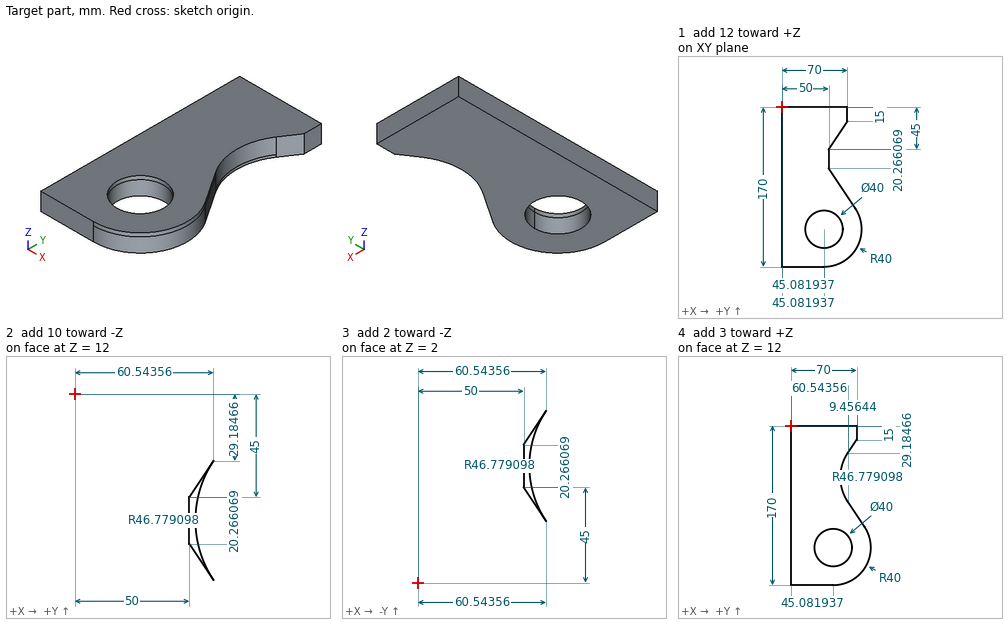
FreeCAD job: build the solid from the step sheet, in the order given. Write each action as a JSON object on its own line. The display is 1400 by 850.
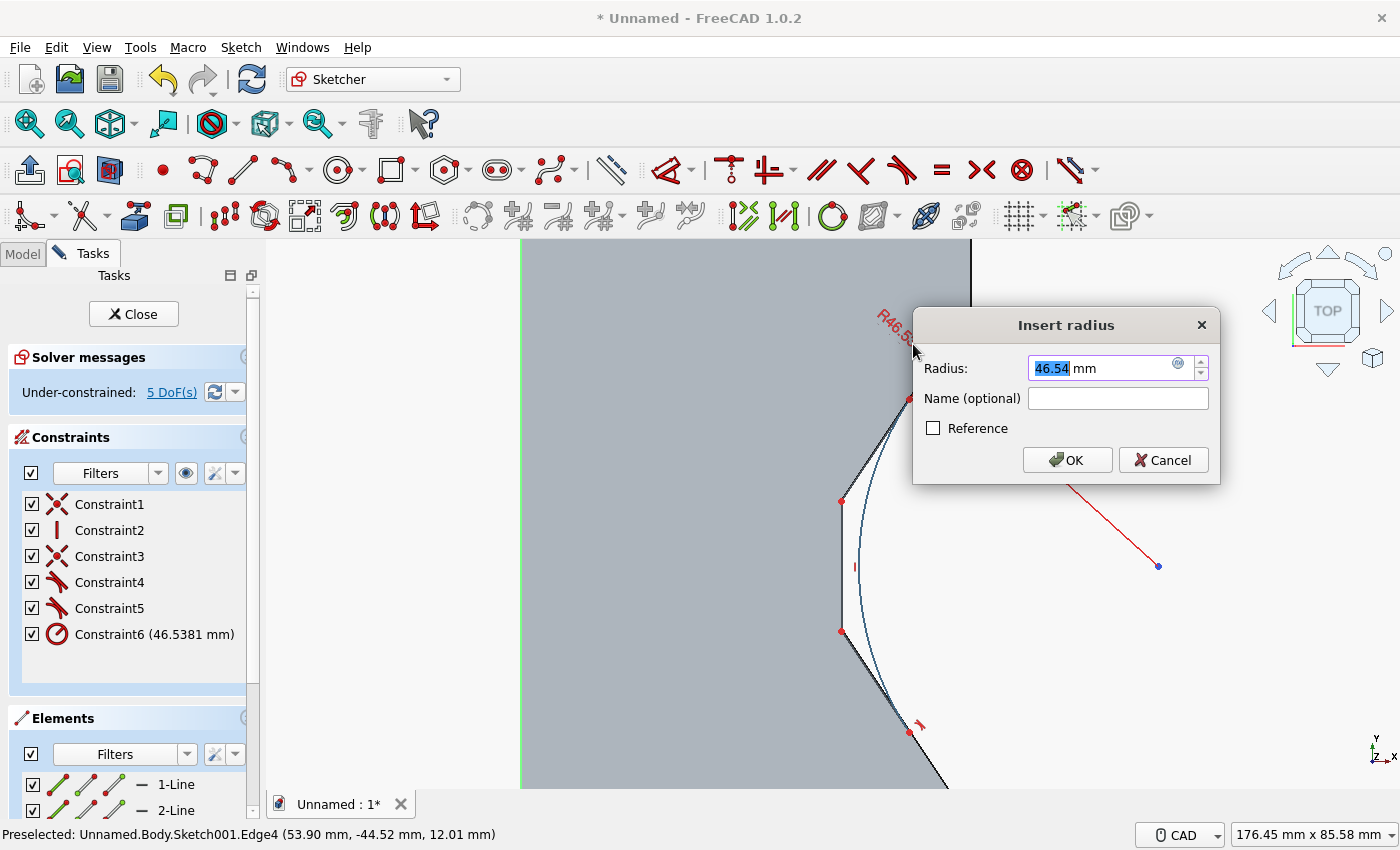
{"action": "type", "text": "46.779098"}
{"action": "key", "text": "Return"}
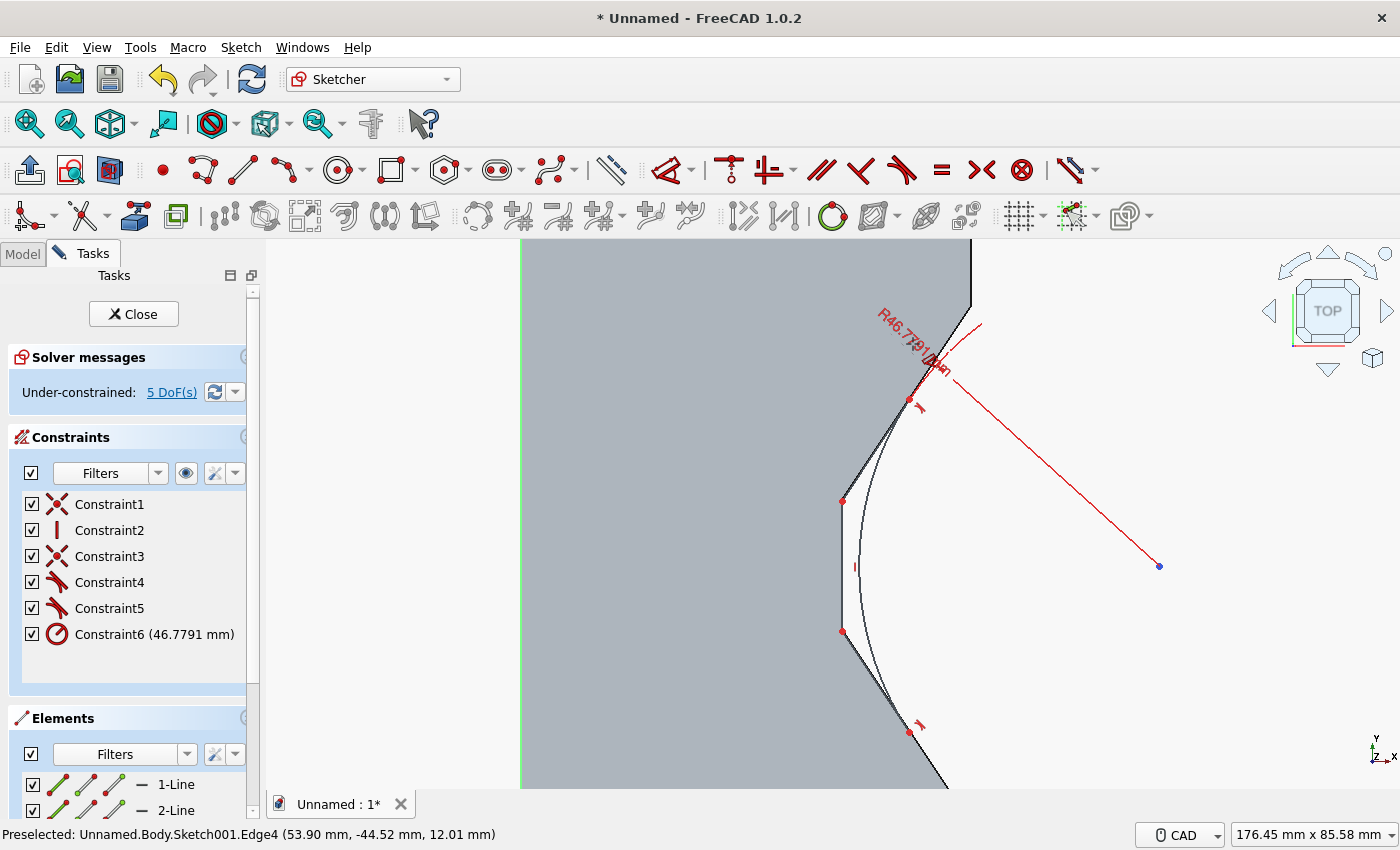
{"action": "left_click", "coordinate": [842, 501]}
{"action": "left_click", "coordinate": [681, 535]}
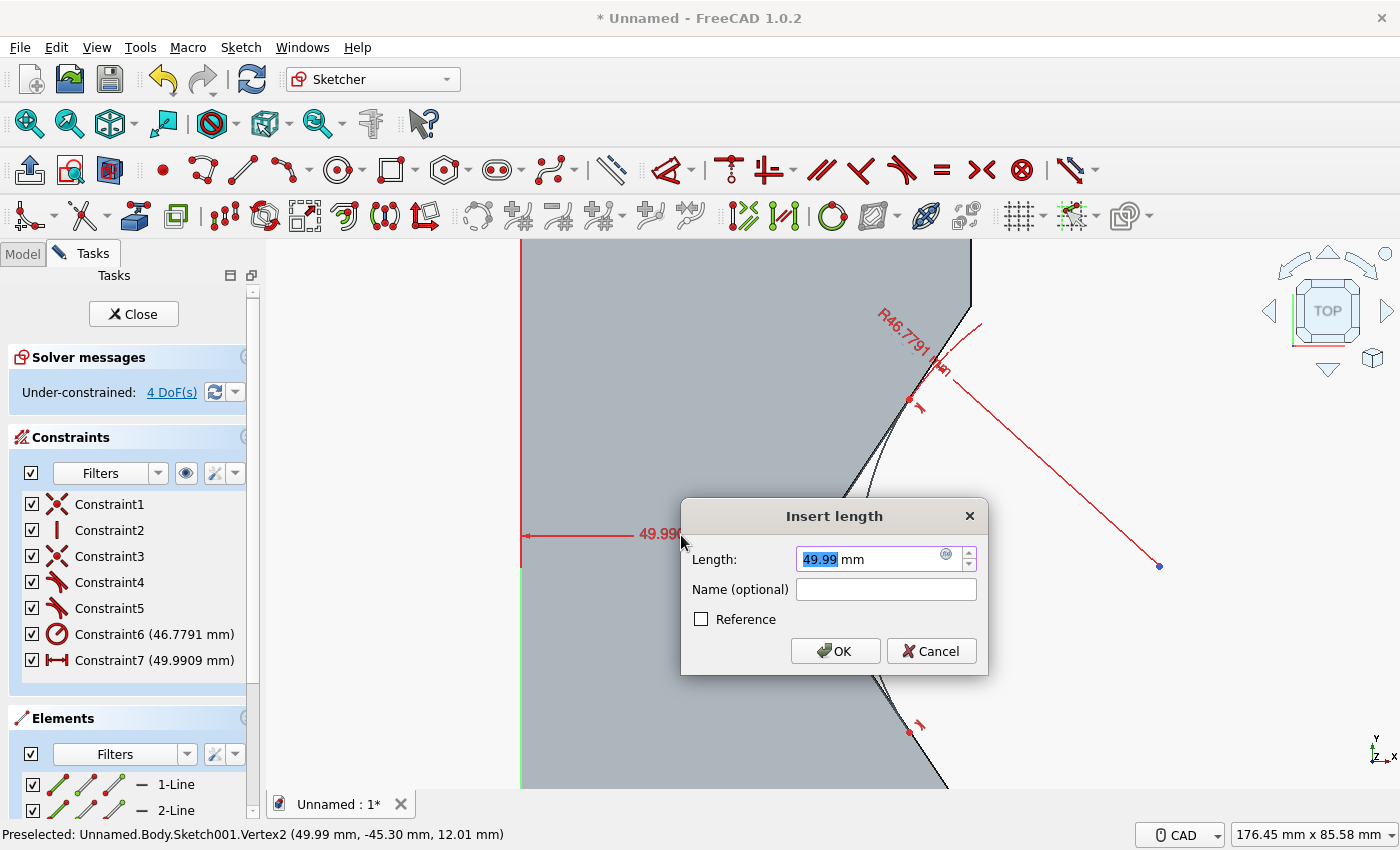
{"action": "type", "text": "50"}
{"action": "key", "text": "Return"}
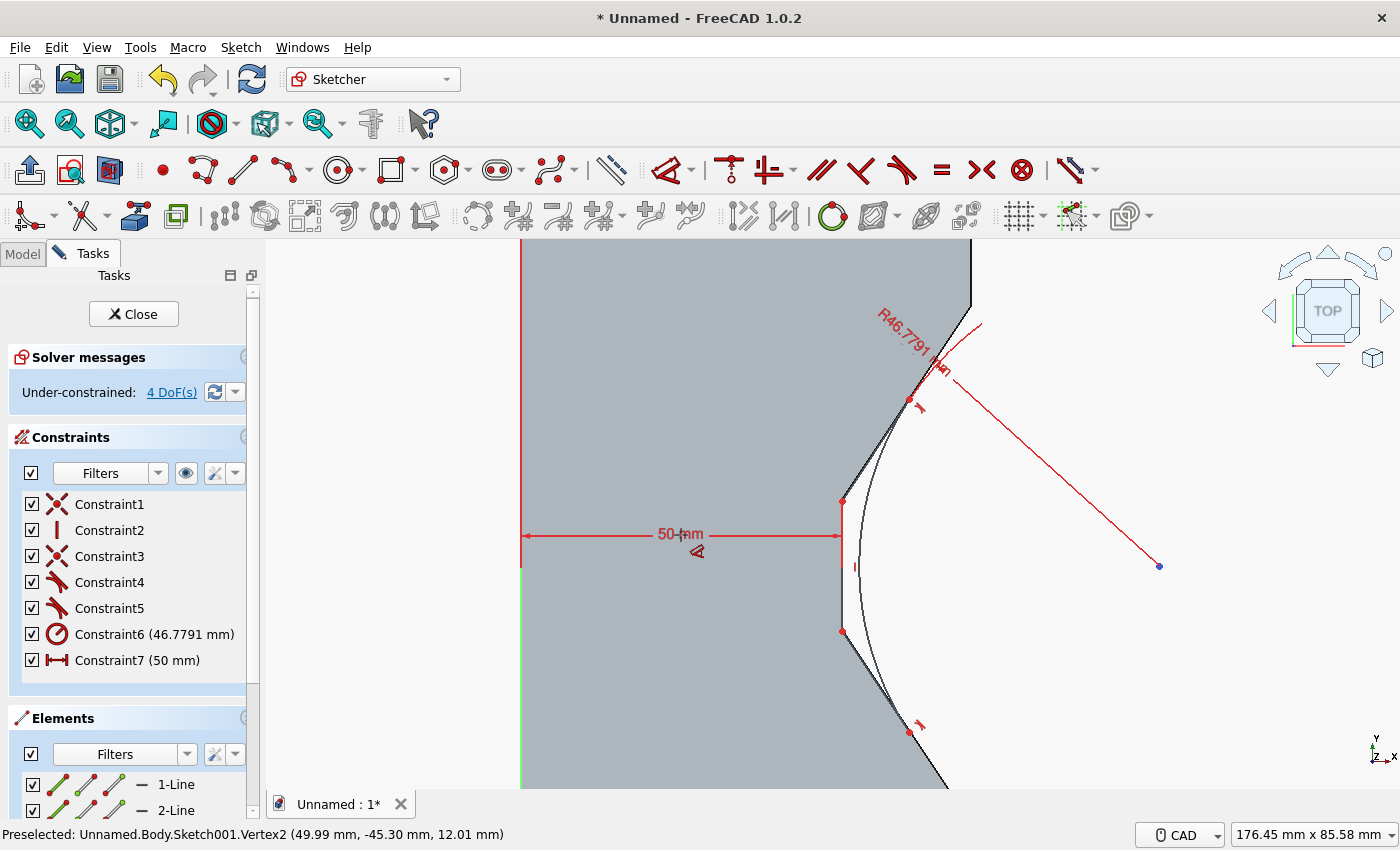
{"action": "left_click", "coordinate": [842, 501]}
{"action": "left_click", "coordinate": [487, 384]}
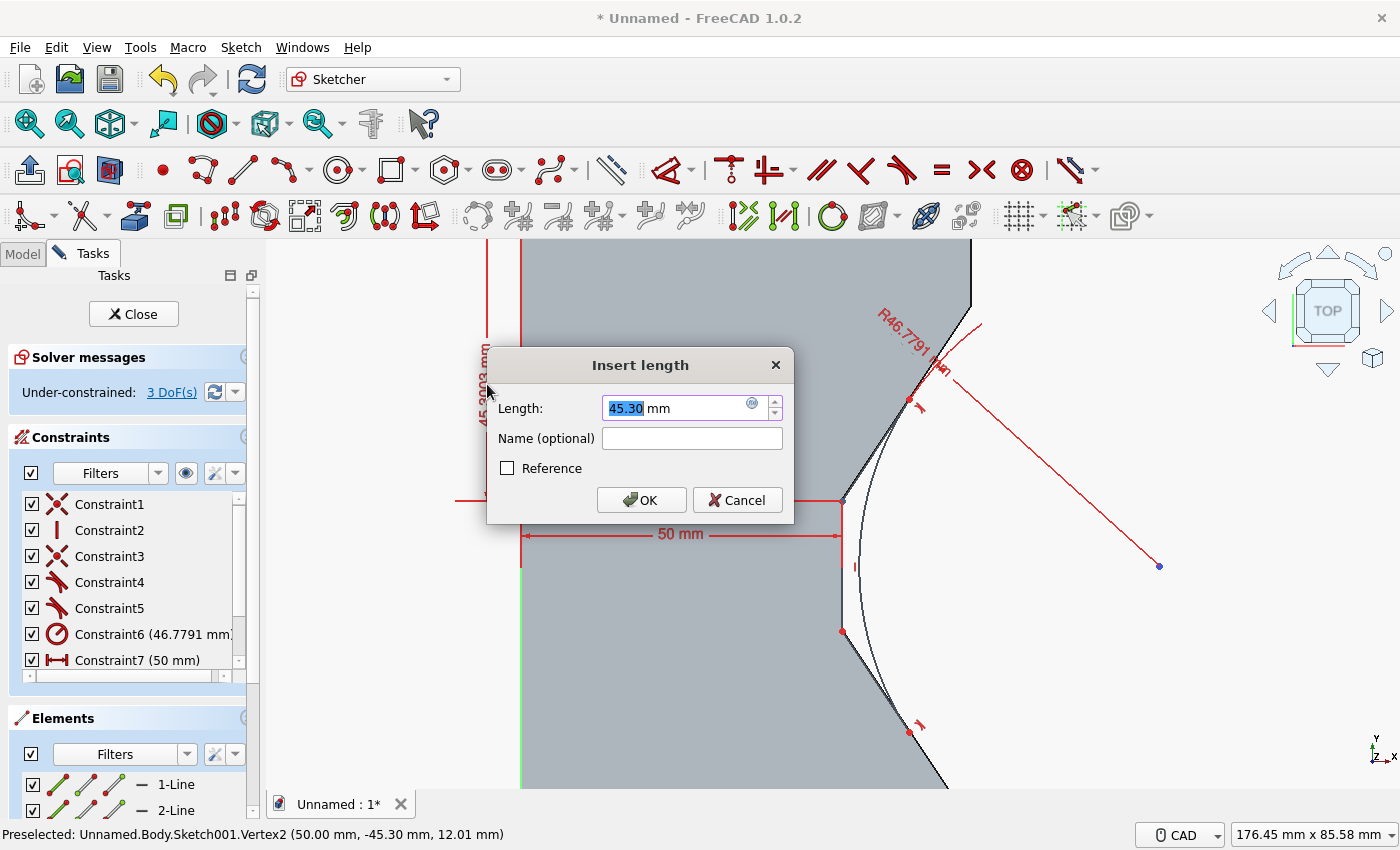
{"action": "type", "text": "45"}
{"action": "key", "text": "Return"}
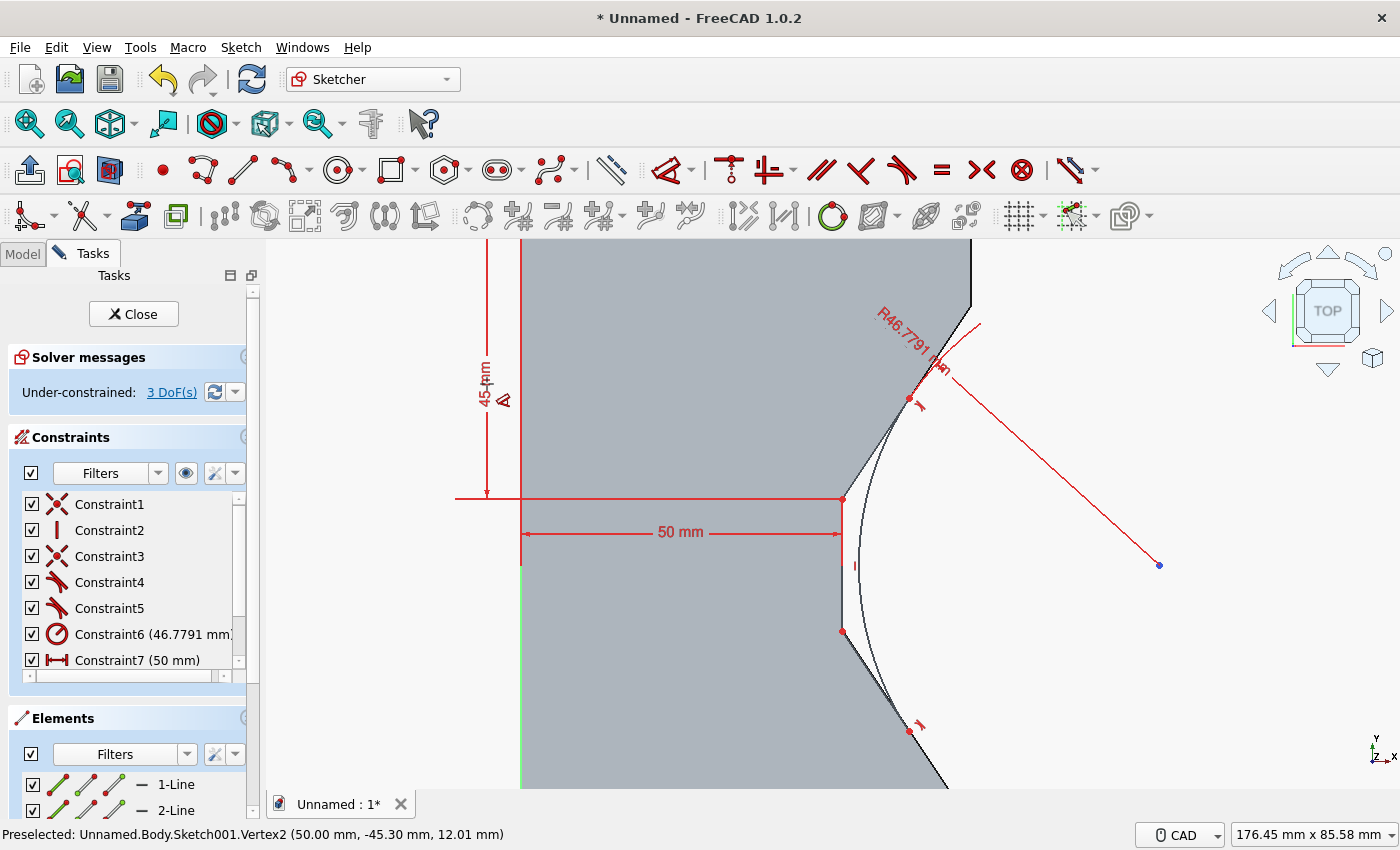
{"action": "left_click", "coordinate": [842, 539]}
{"action": "left_click", "coordinate": [876, 565]}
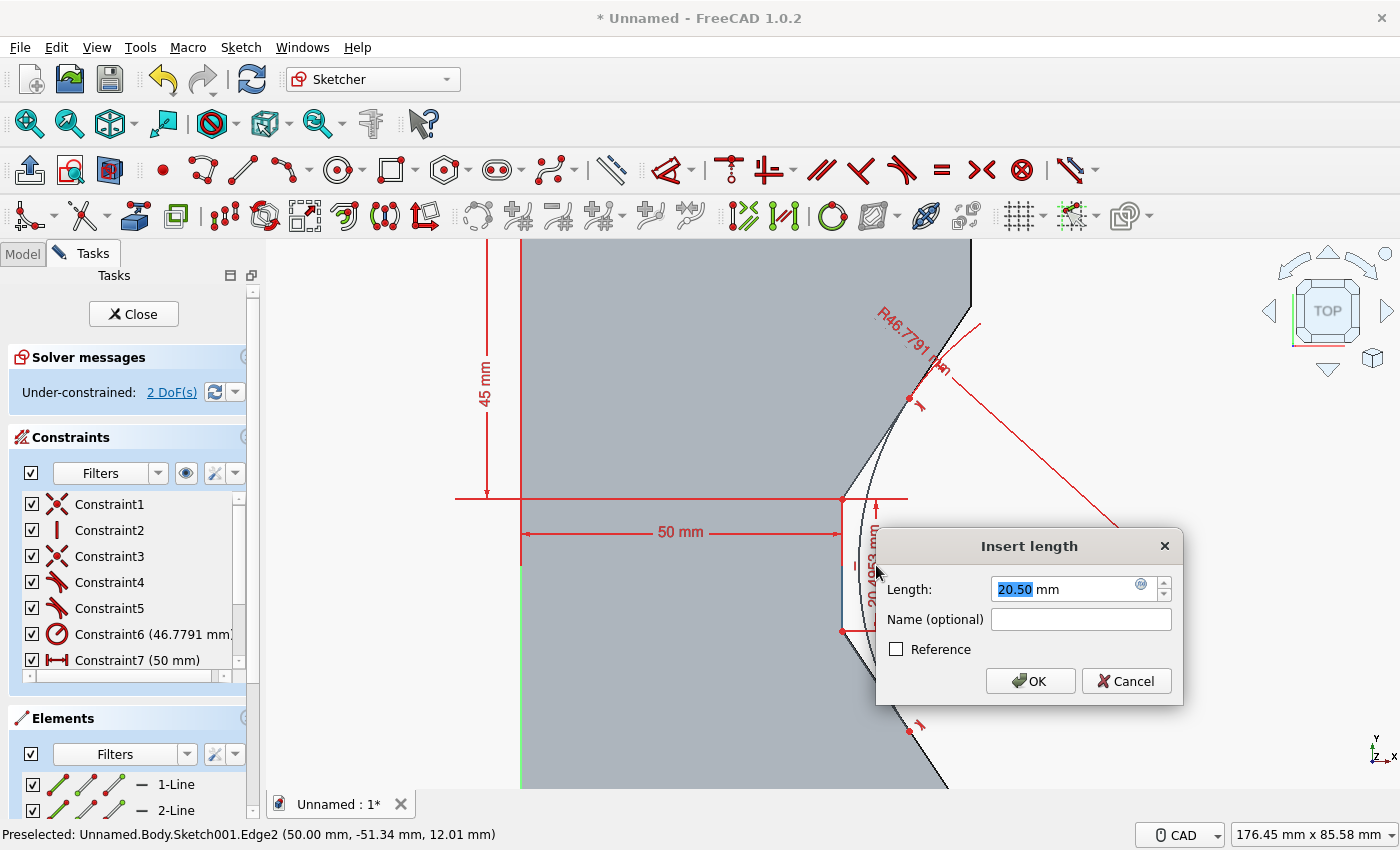
{"action": "type", "text": "20.266069"}
{"action": "key", "text": "Return"}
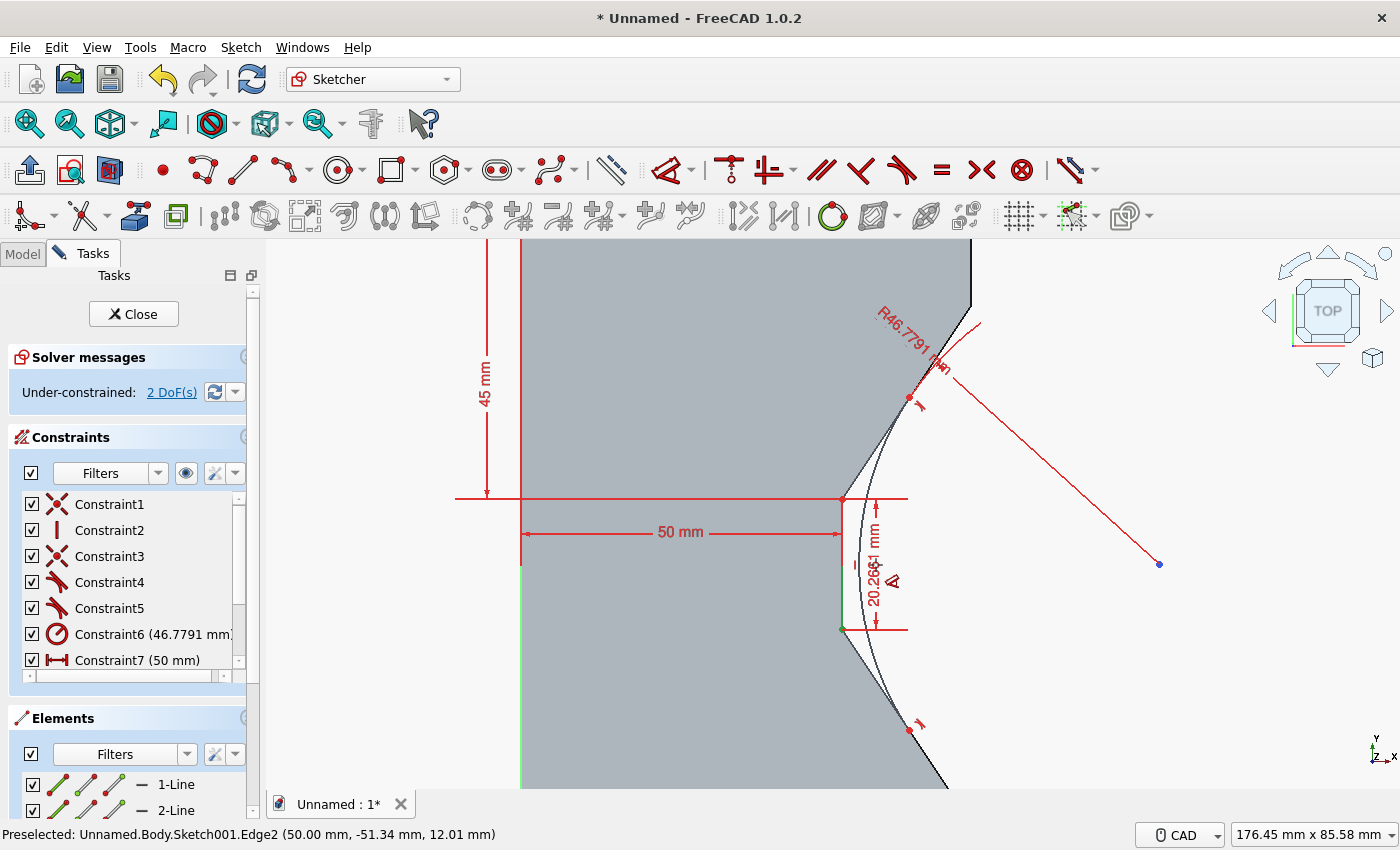
{"action": "left_click", "coordinate": [909, 398]}
{"action": "left_click", "coordinate": [715, 432]}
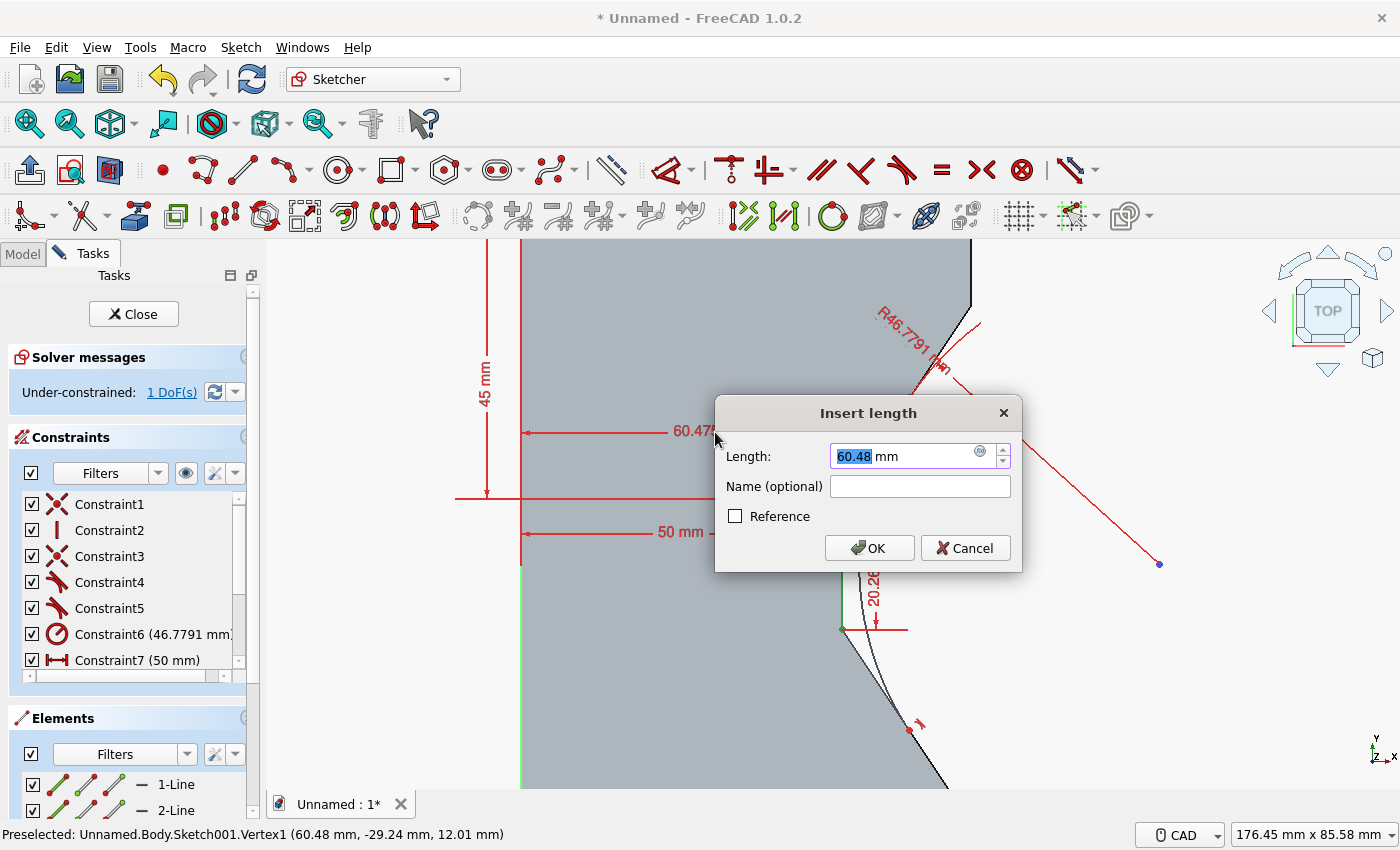
{"action": "type", "text": "60.54356"}
{"action": "key", "text": "Return"}